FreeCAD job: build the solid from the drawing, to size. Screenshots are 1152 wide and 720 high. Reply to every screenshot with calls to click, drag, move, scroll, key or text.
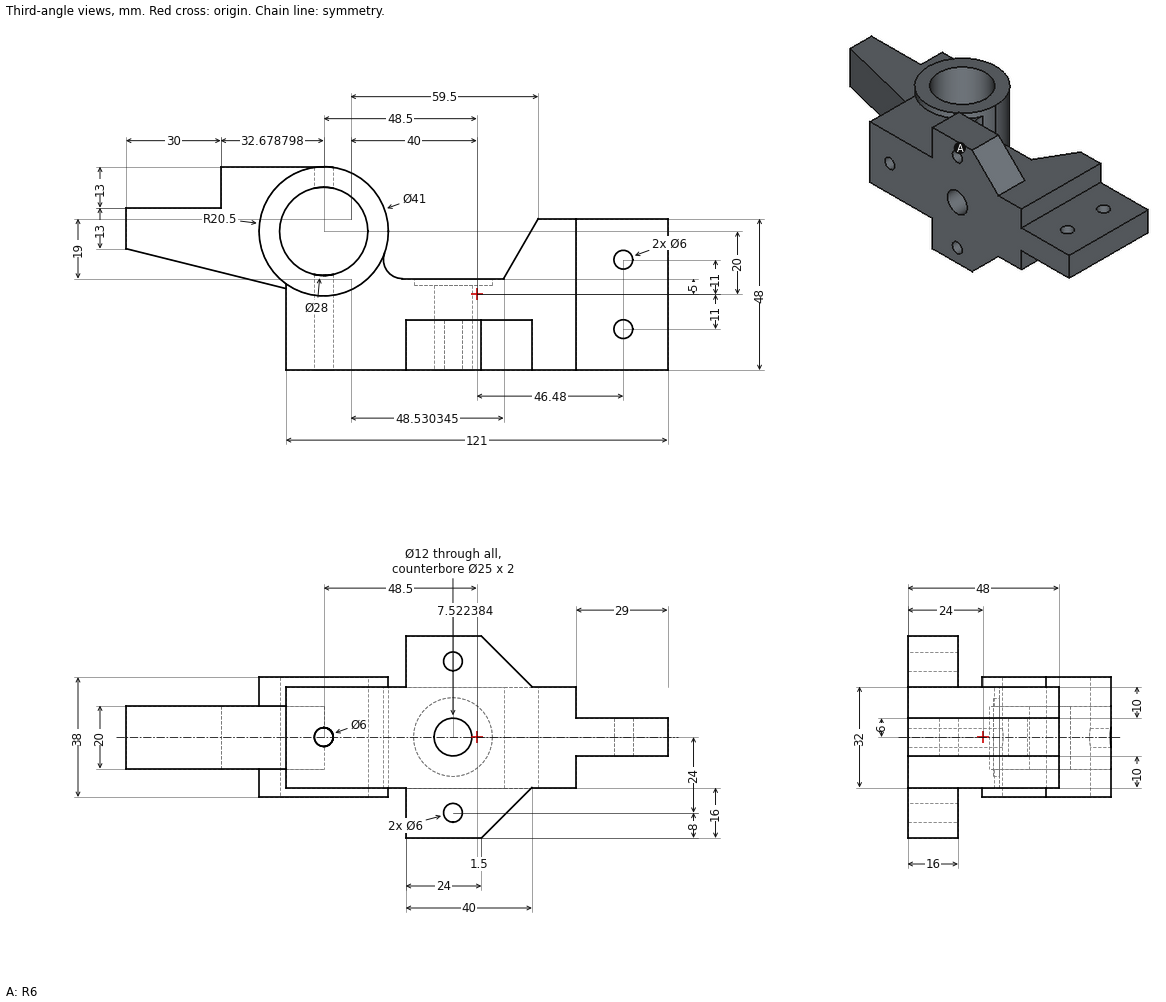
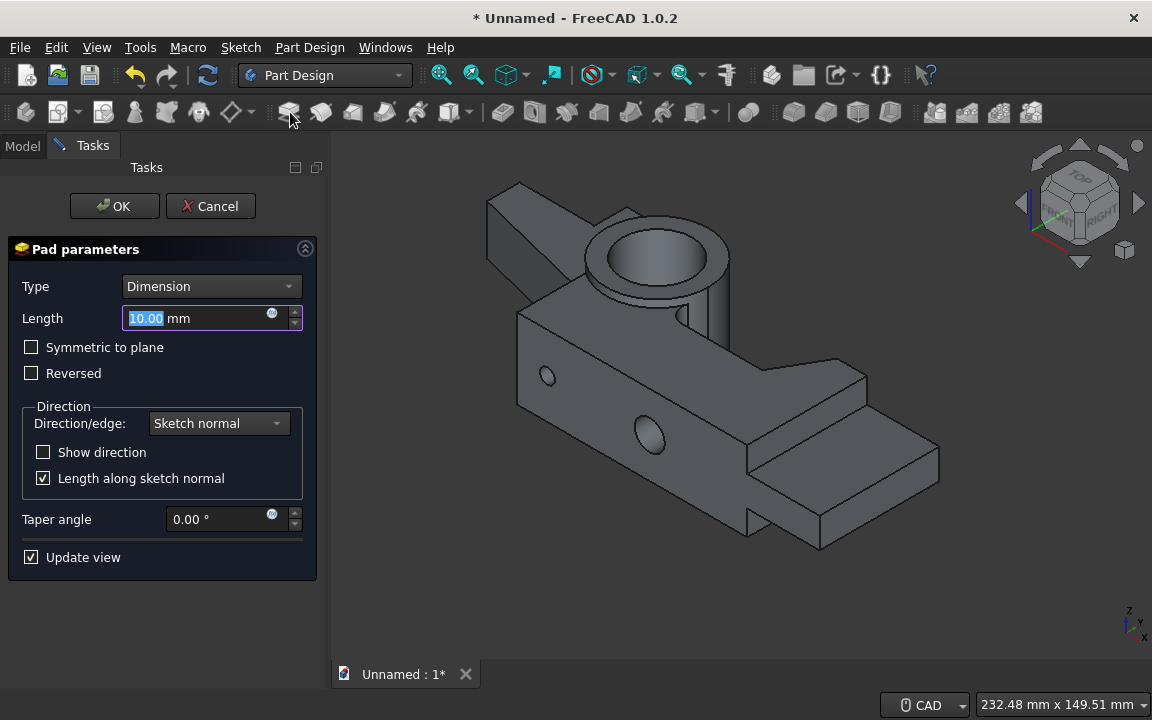
text(16)
key(Tab)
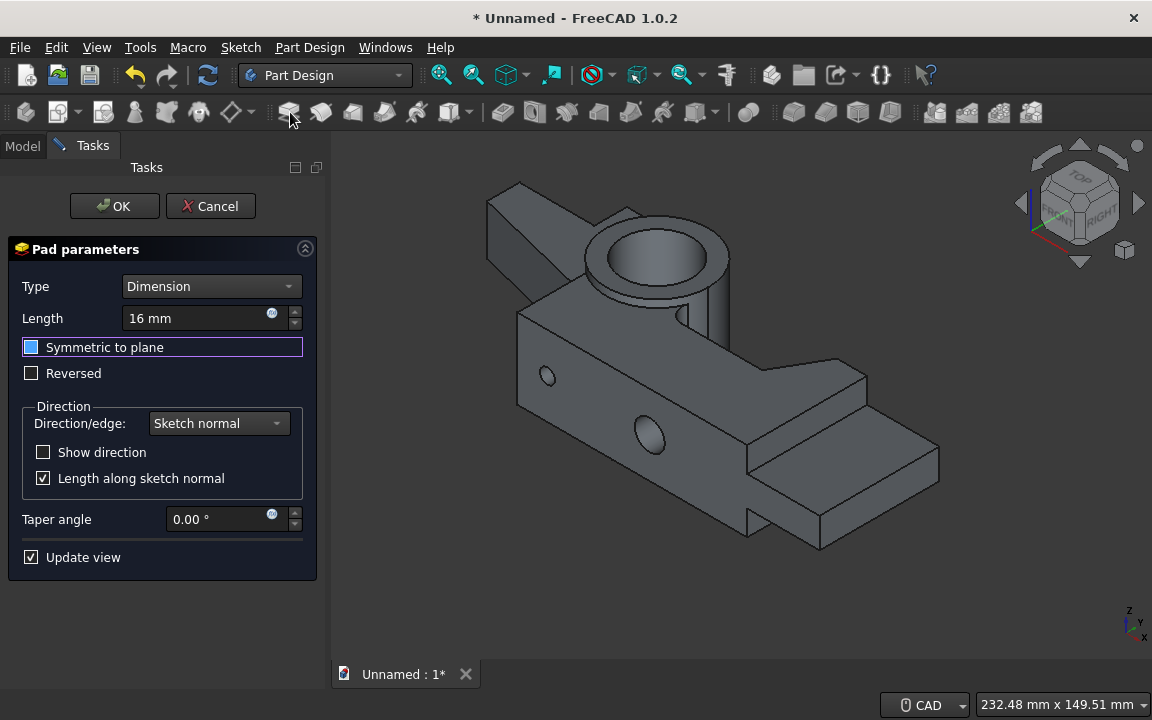
click(30, 373)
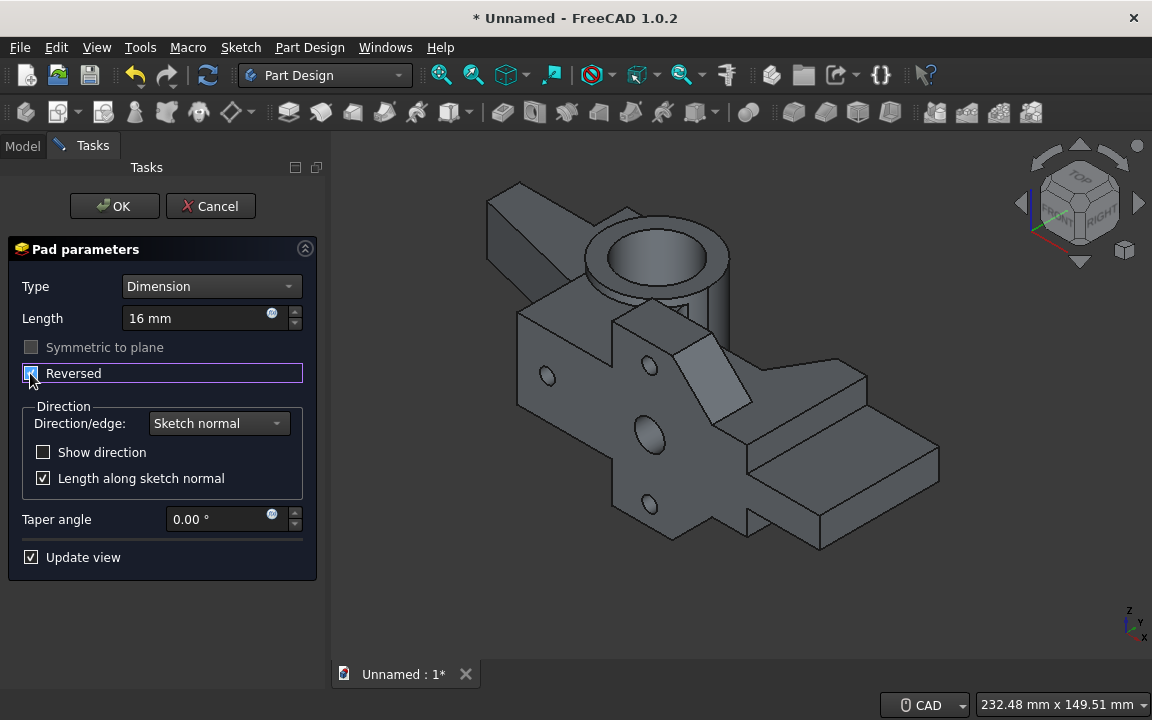
click(115, 206)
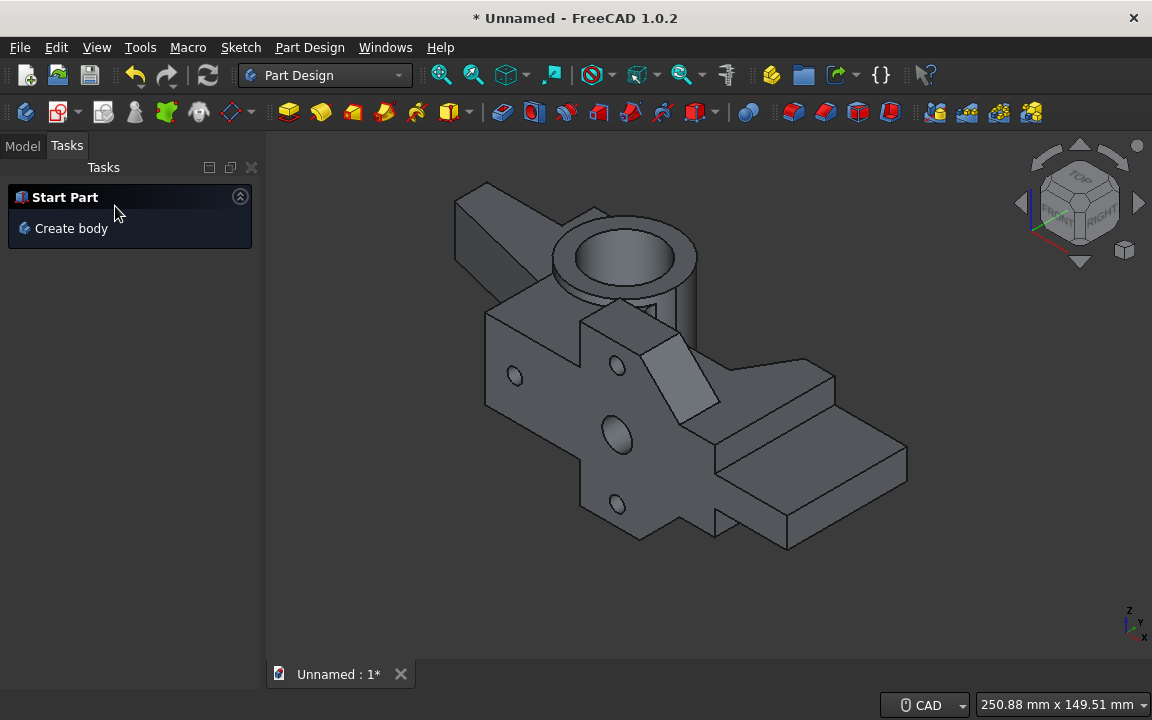
click(442, 76)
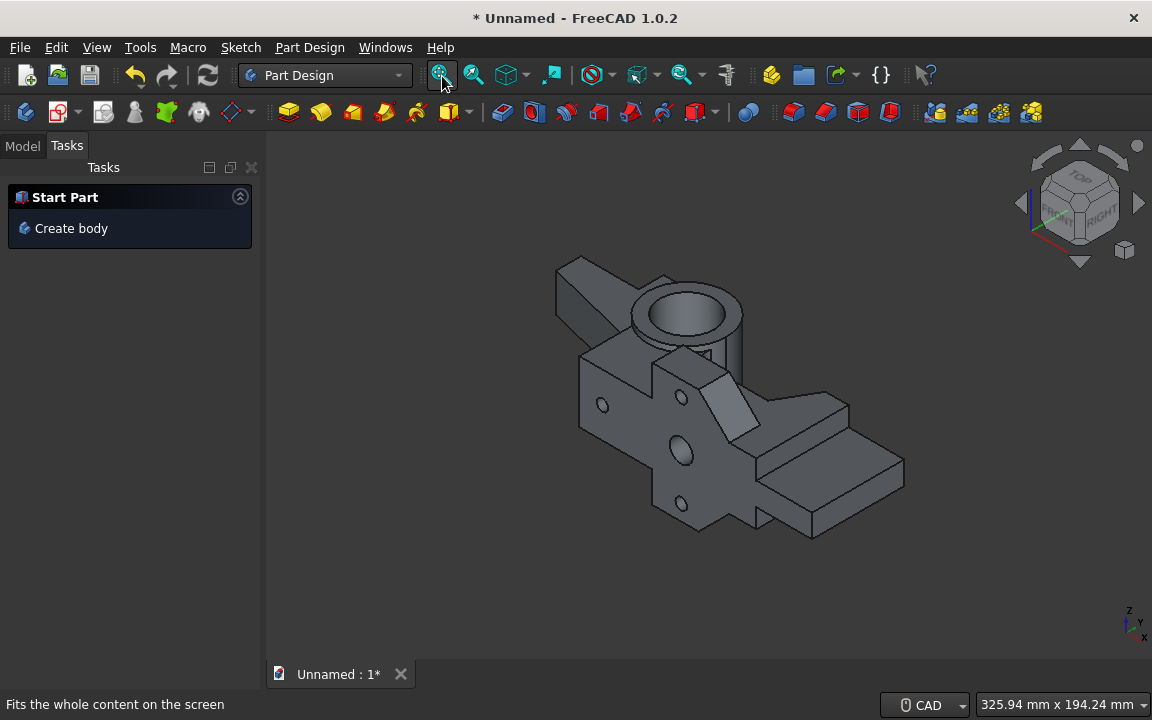
click(843, 461)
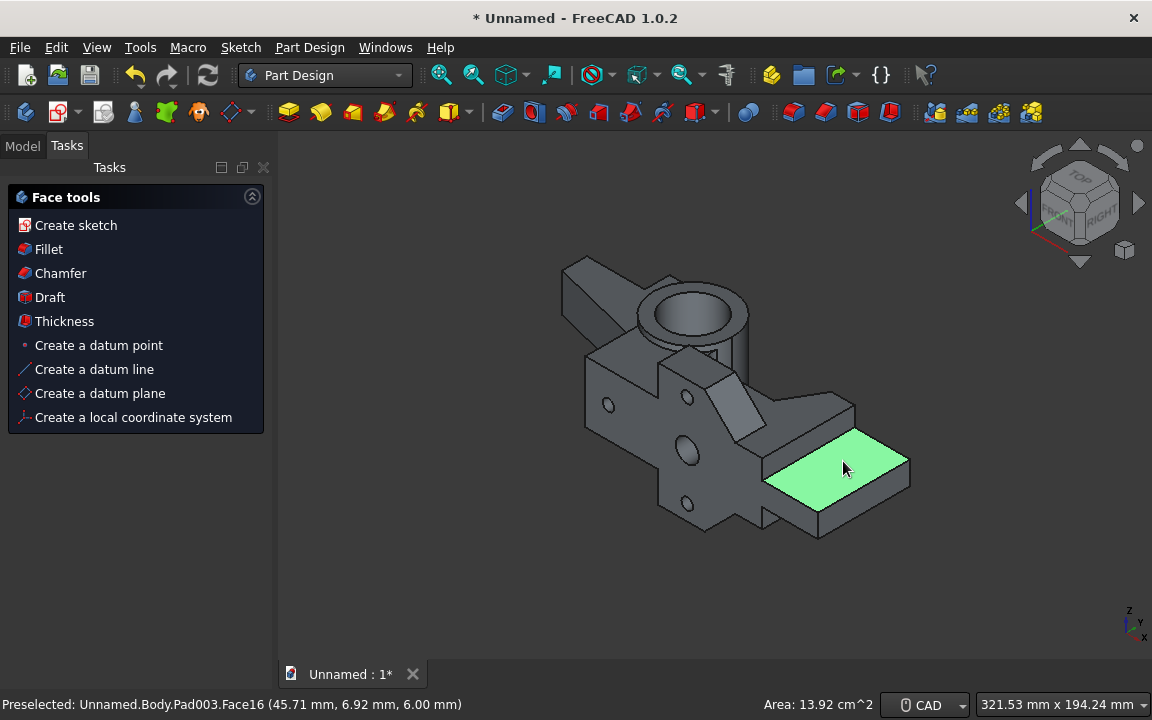
click(58, 112)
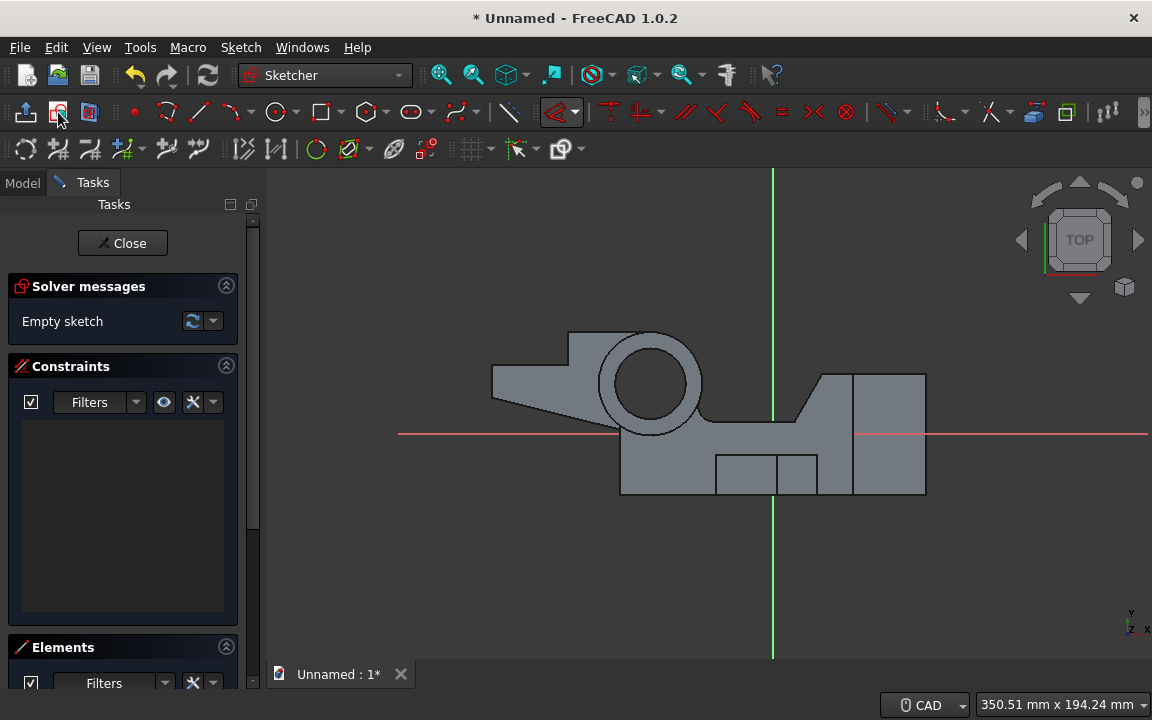
scroll(899, 441, up, 7)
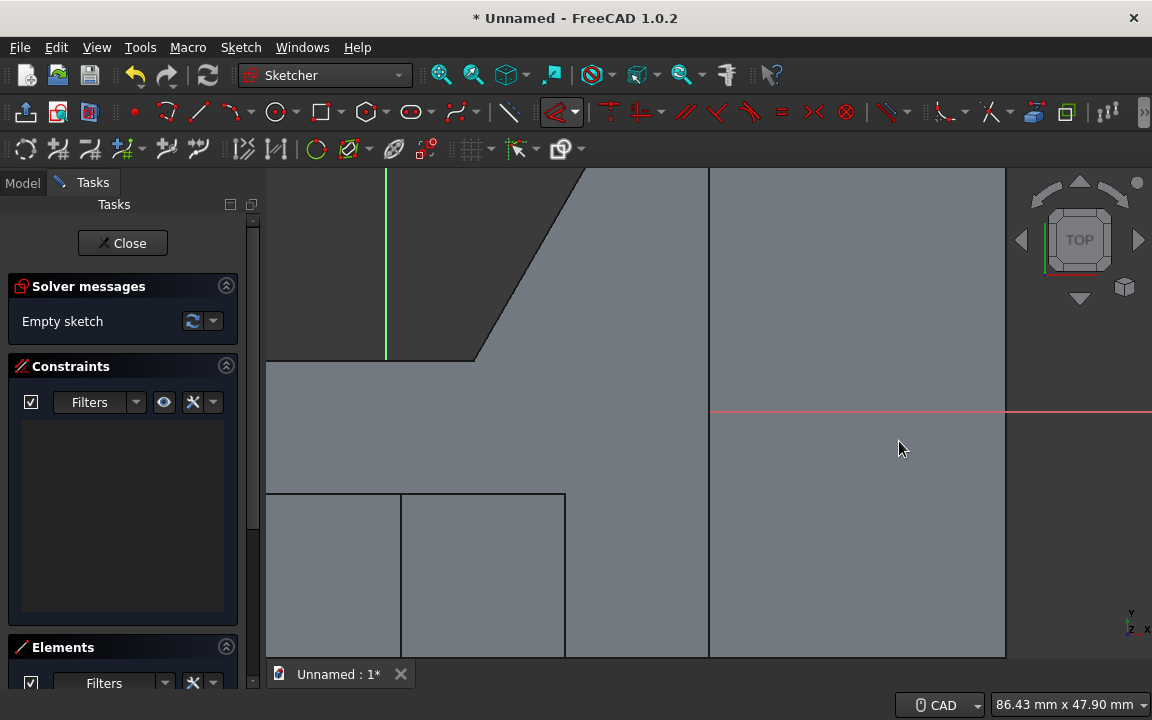
click(276, 112)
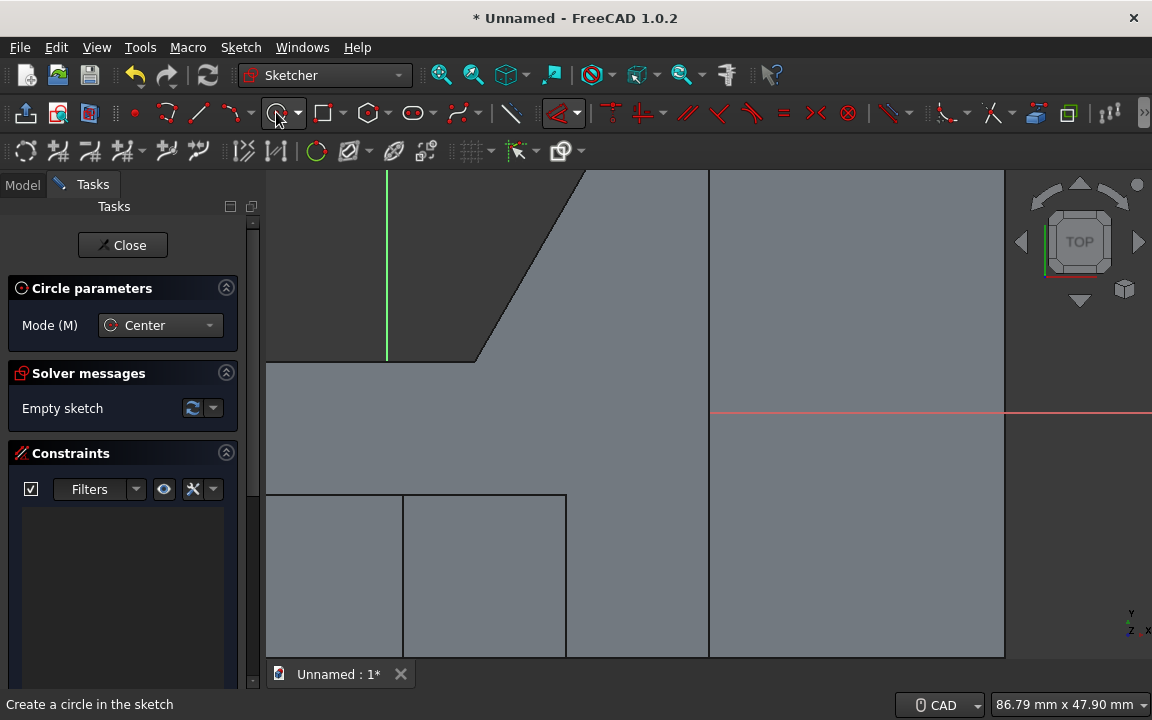
click(862, 301)
move(884, 279)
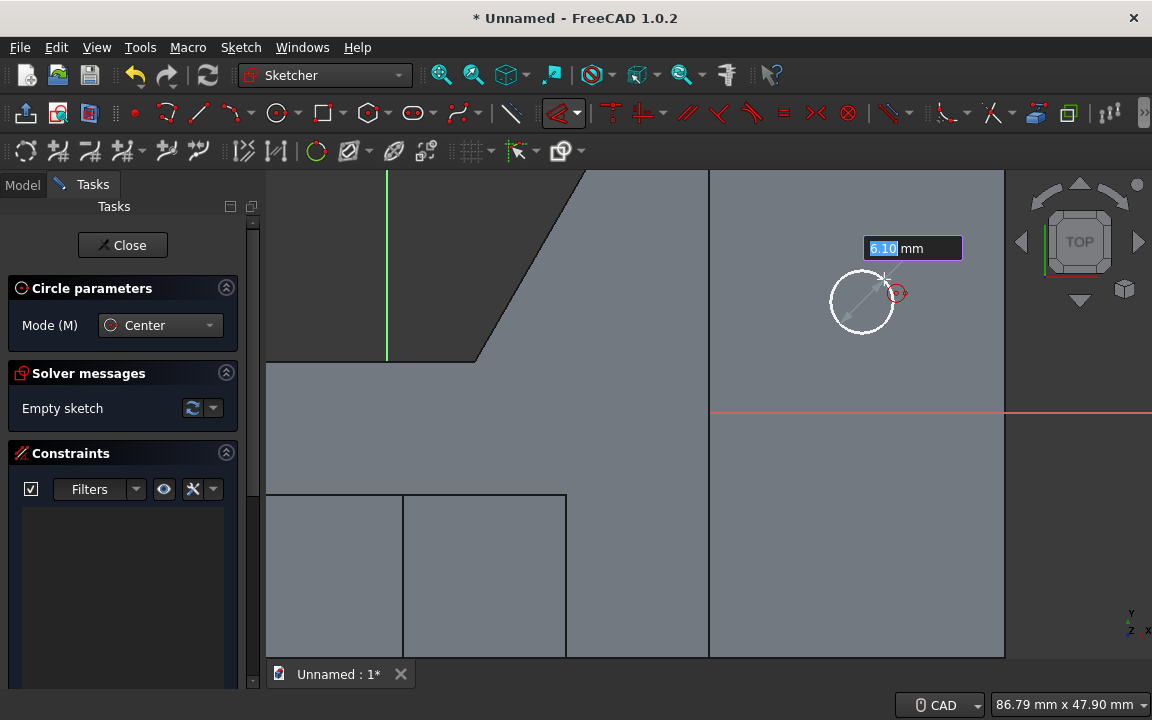
text(6)
key(Return)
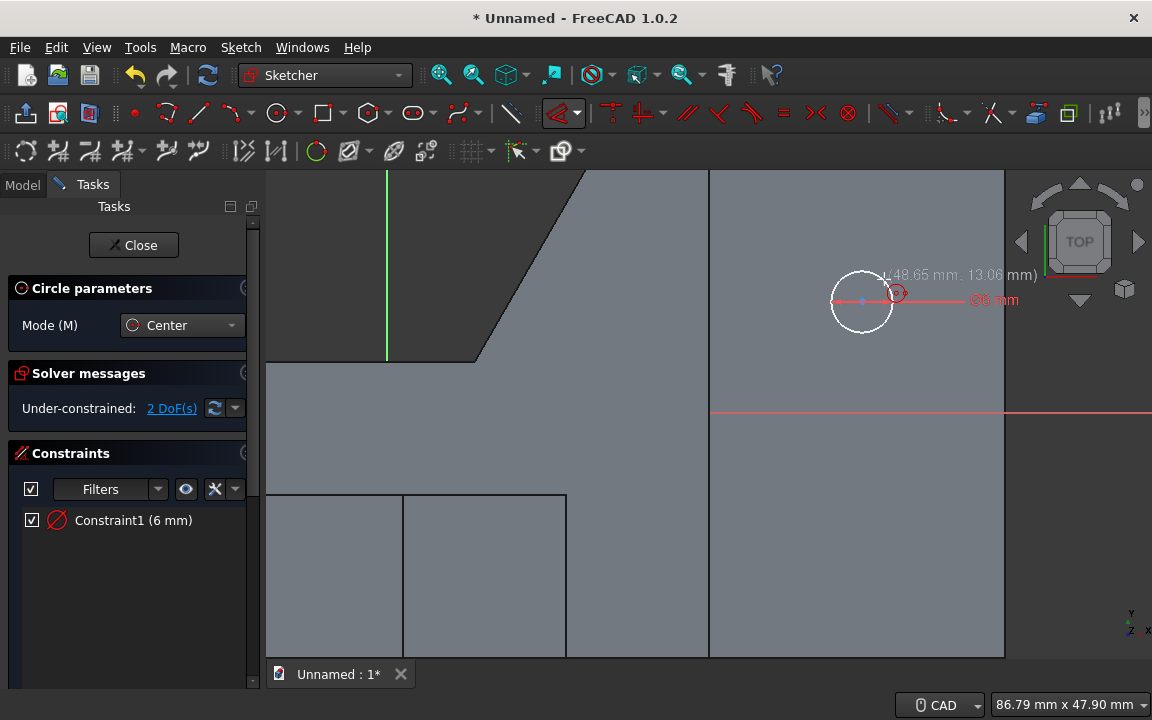
click(862, 526)
move(884, 504)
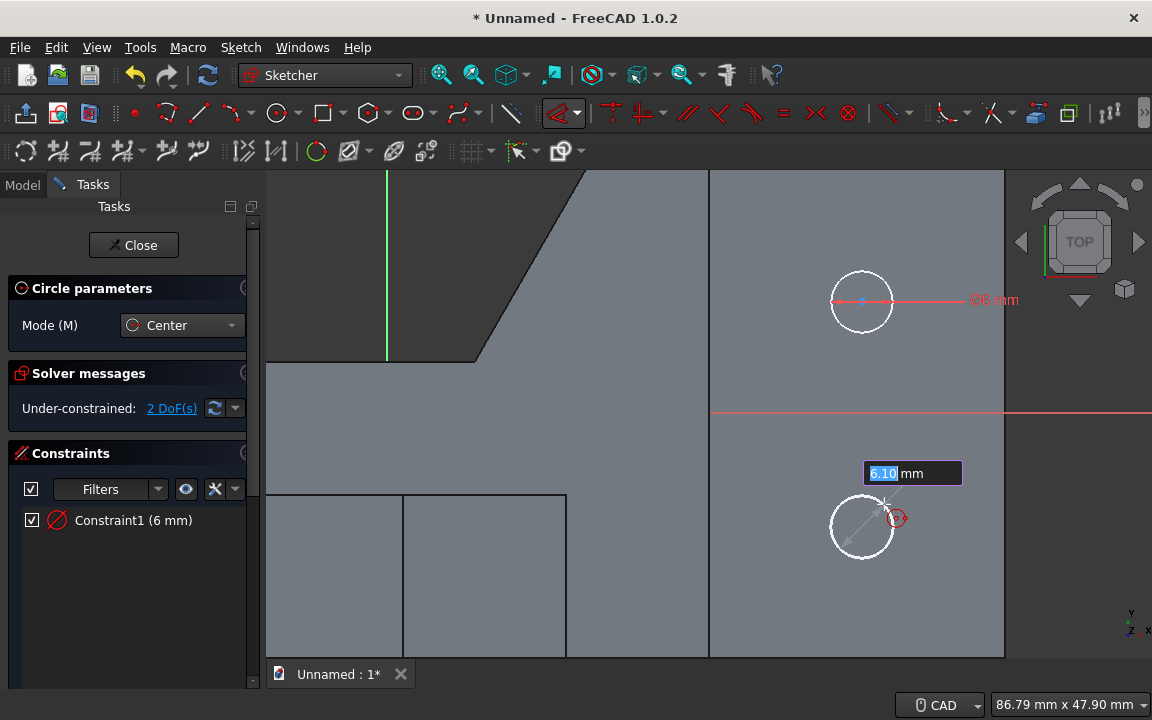
text(6)
key(Return)
key(Escape)